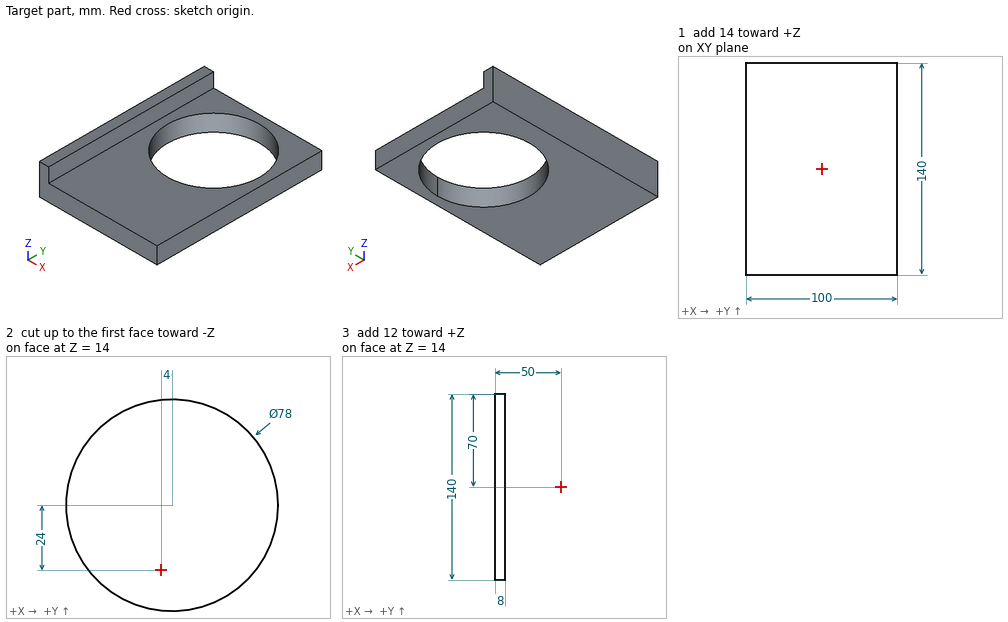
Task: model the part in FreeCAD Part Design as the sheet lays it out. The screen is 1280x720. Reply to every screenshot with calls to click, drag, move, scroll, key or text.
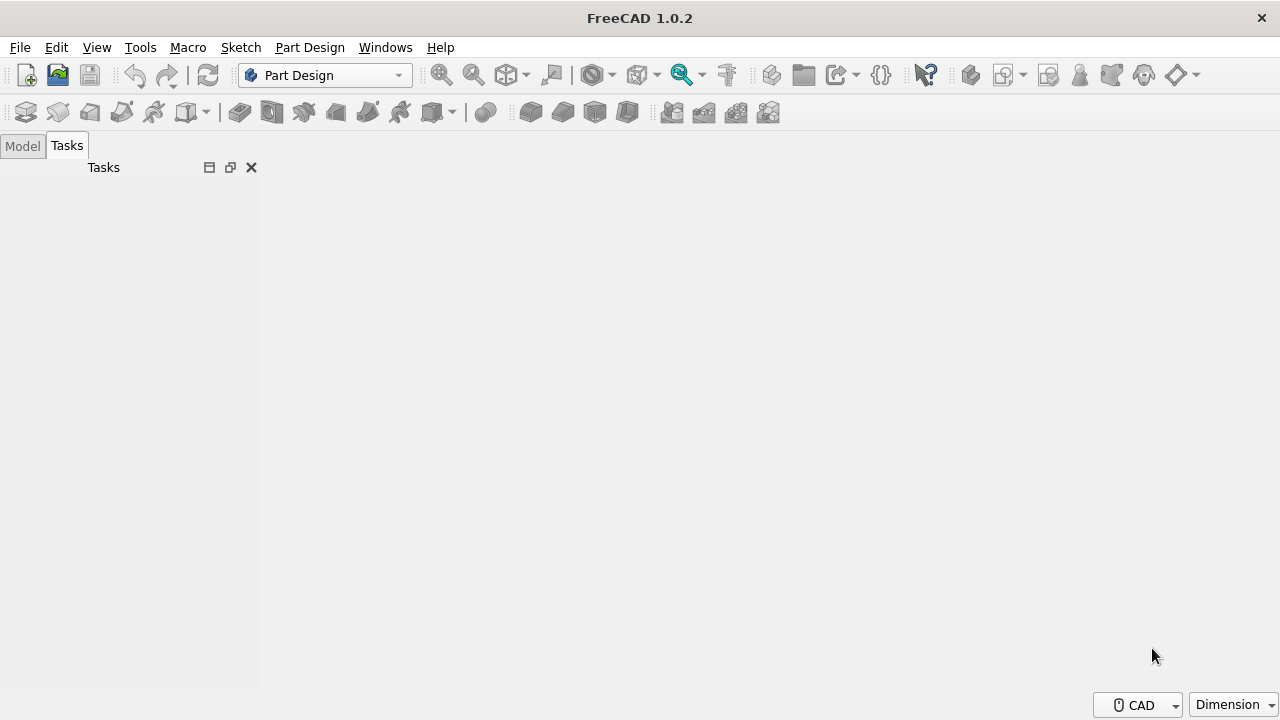
key(ctrl+n)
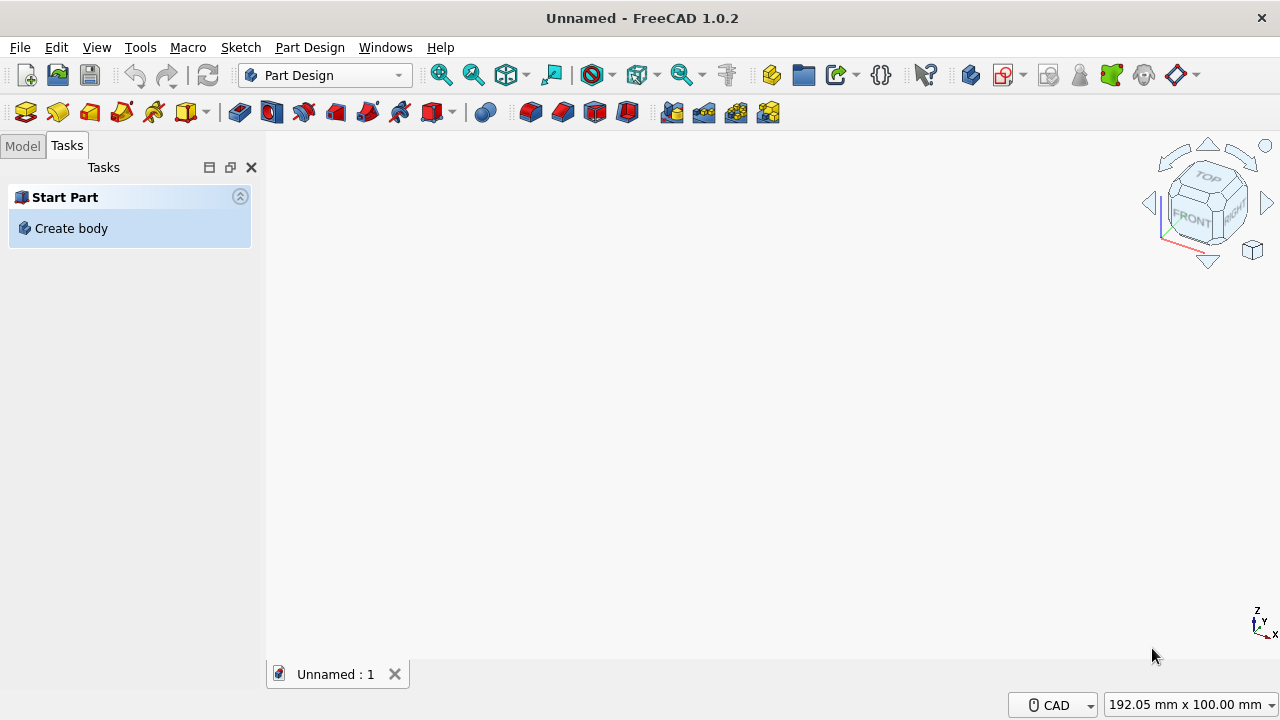
click(1004, 76)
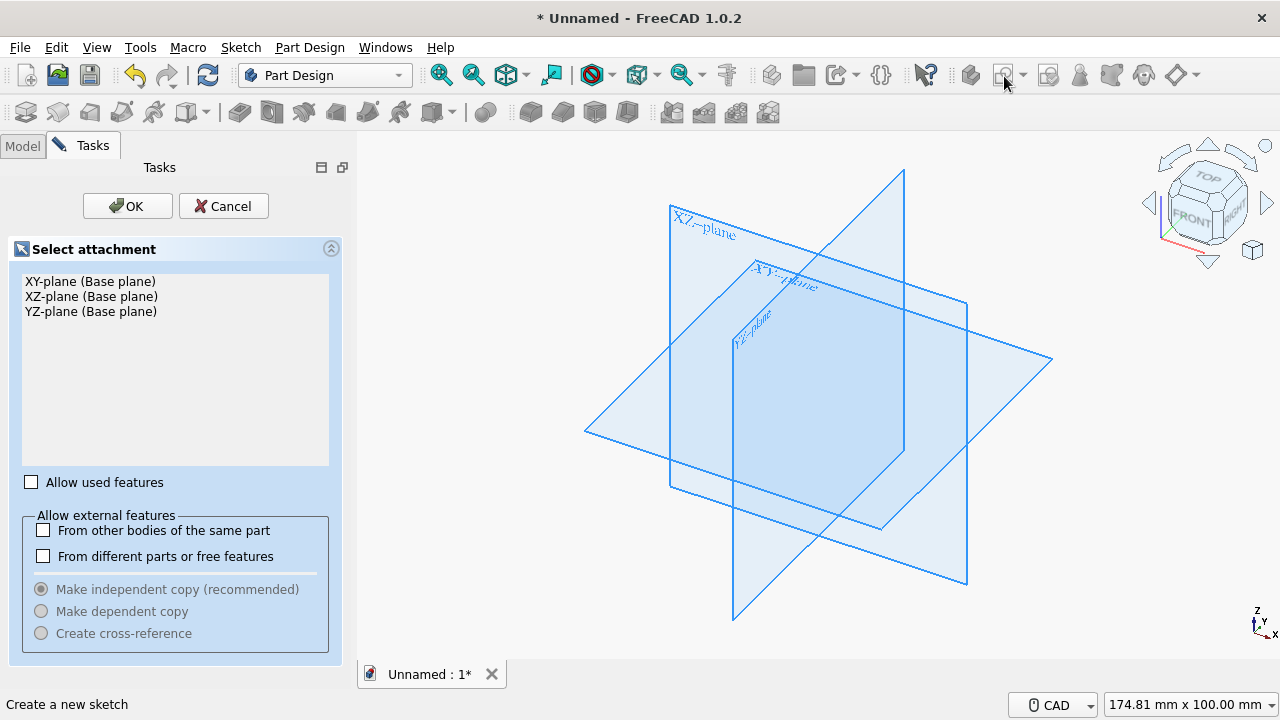
click(82, 282)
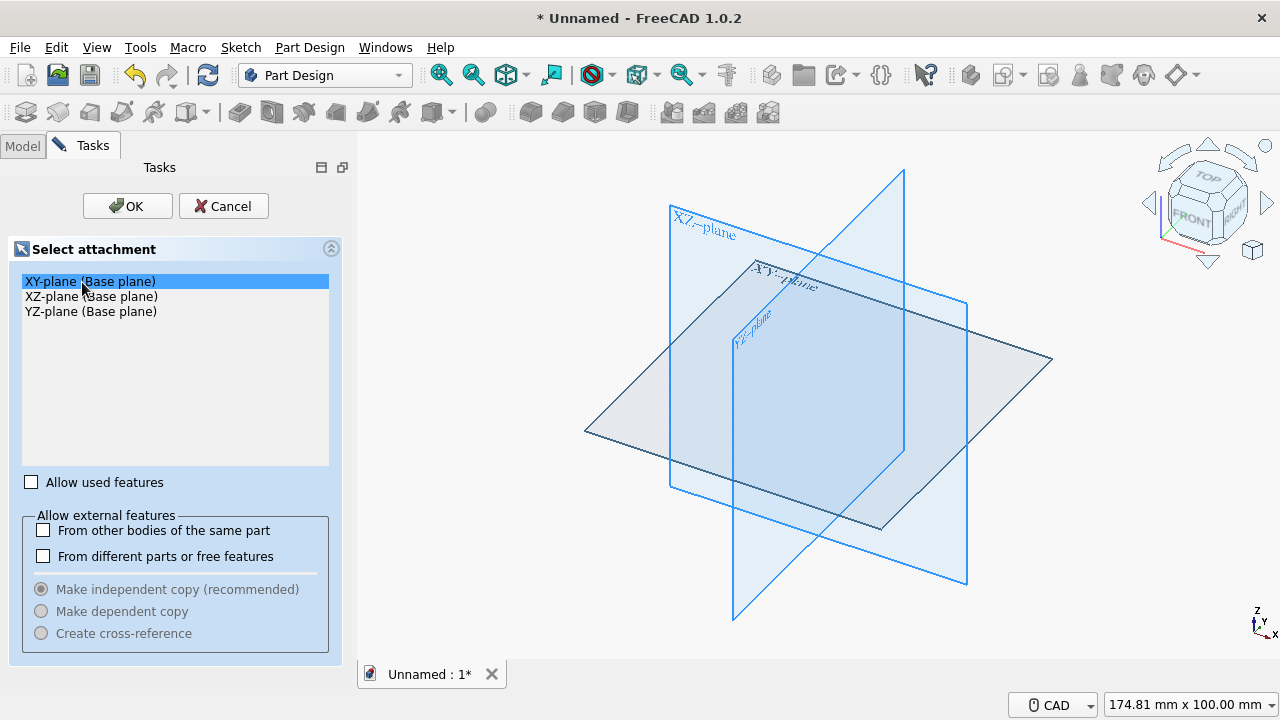
click(128, 206)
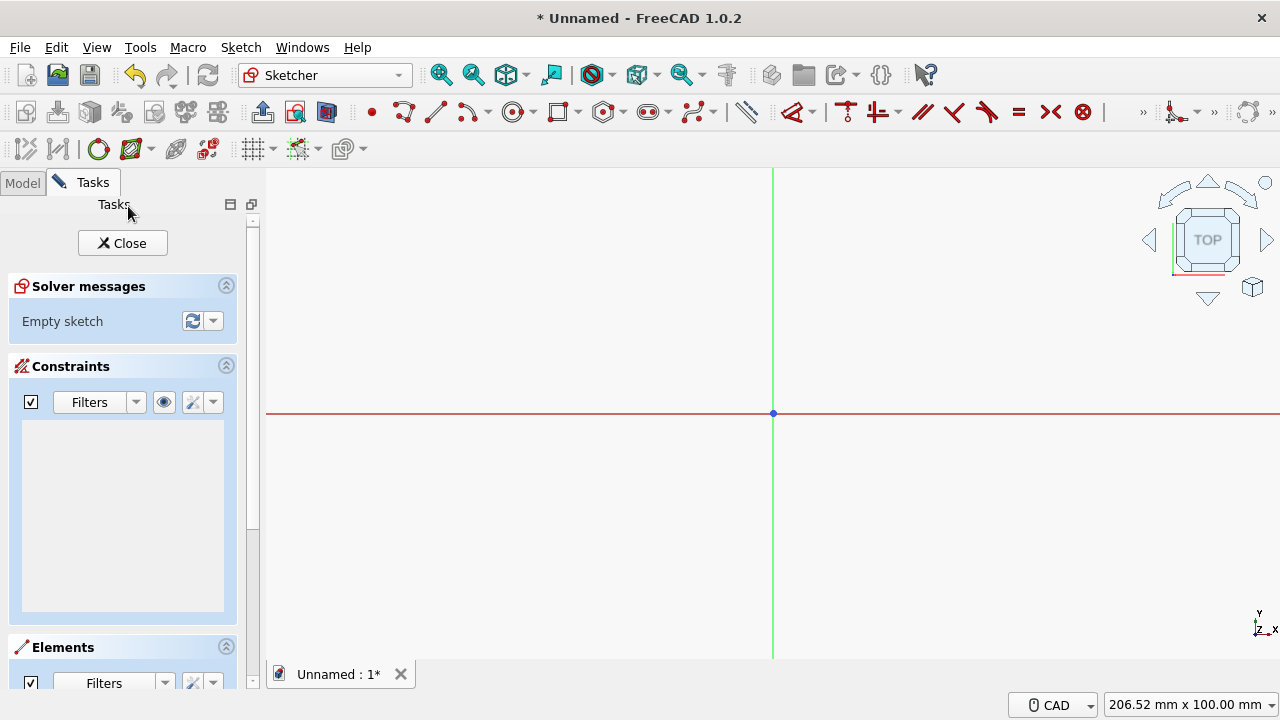
scroll(649, 414, down, 4)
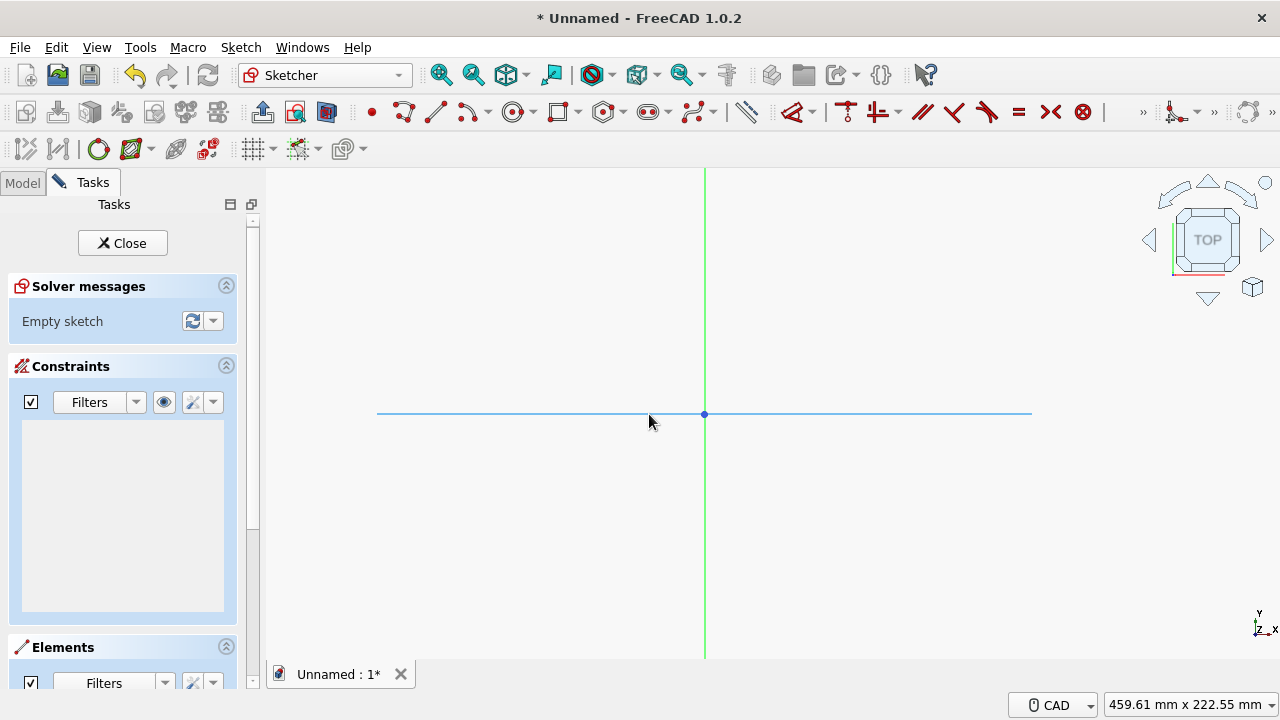
click(580, 112)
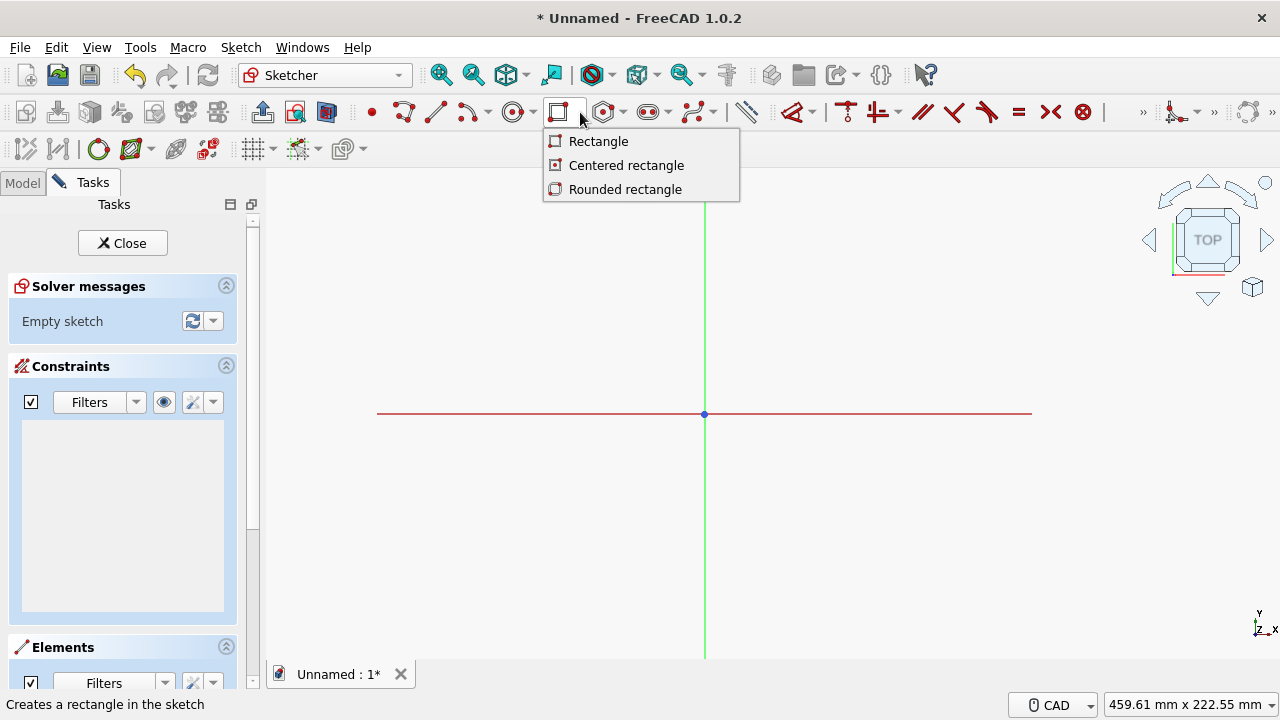
click(642, 165)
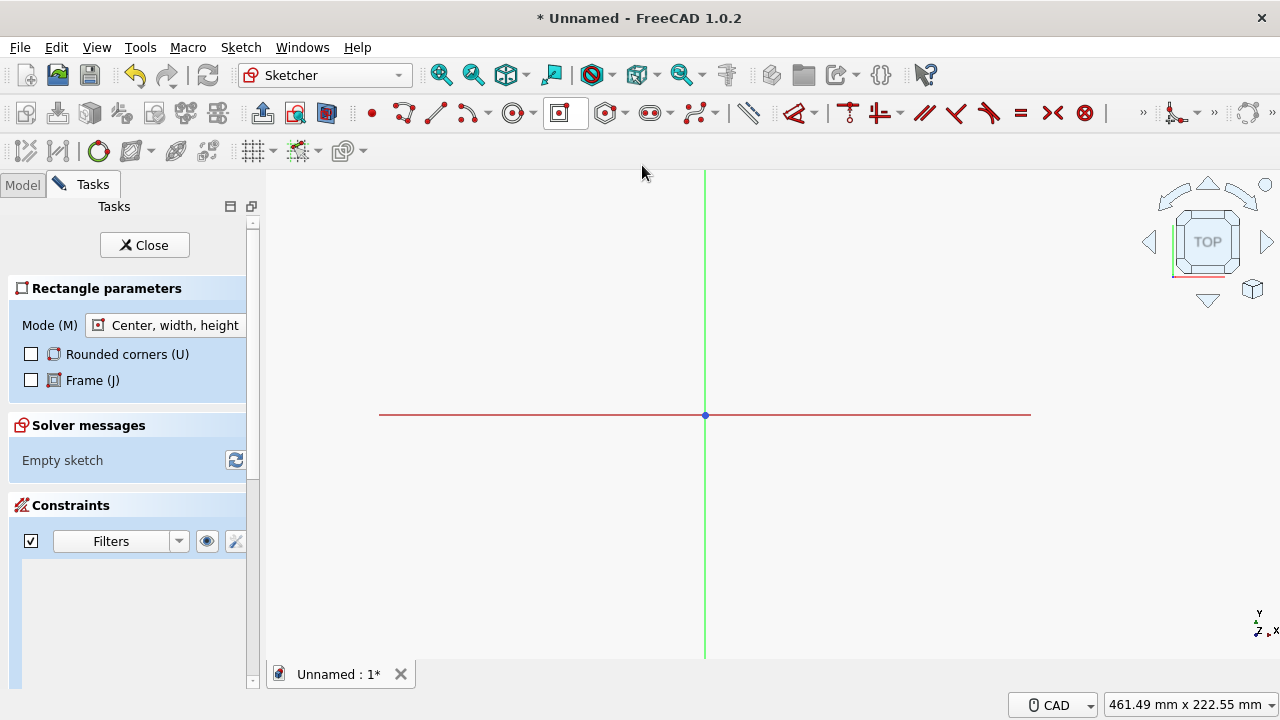
click(705, 415)
move(815, 261)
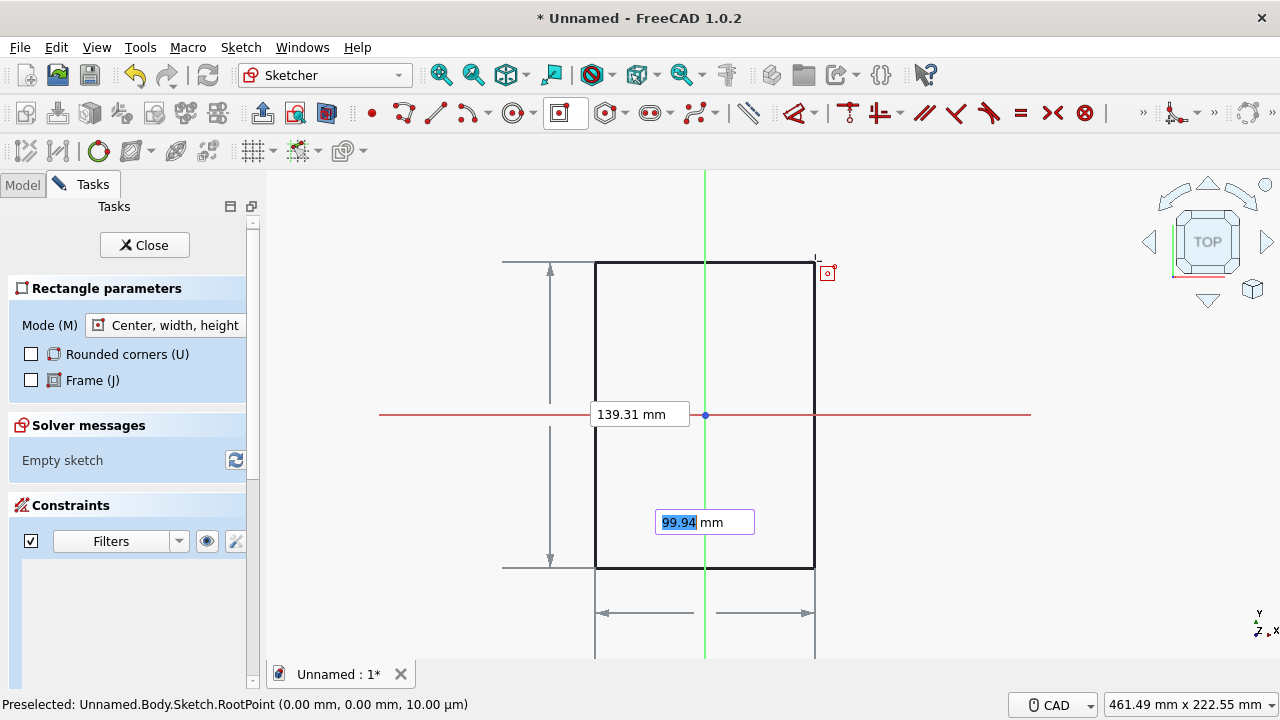
text(100)
key(Tab)
text(140)
key(Return)
key(Escape)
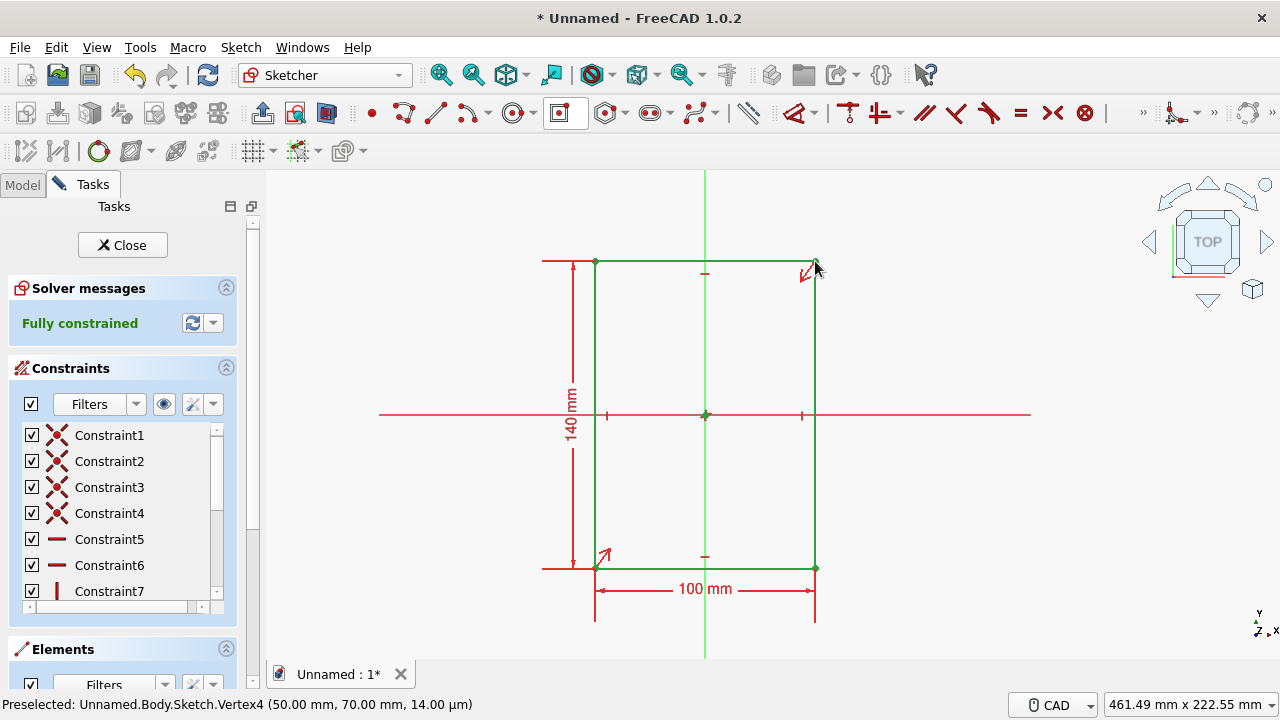
click(123, 245)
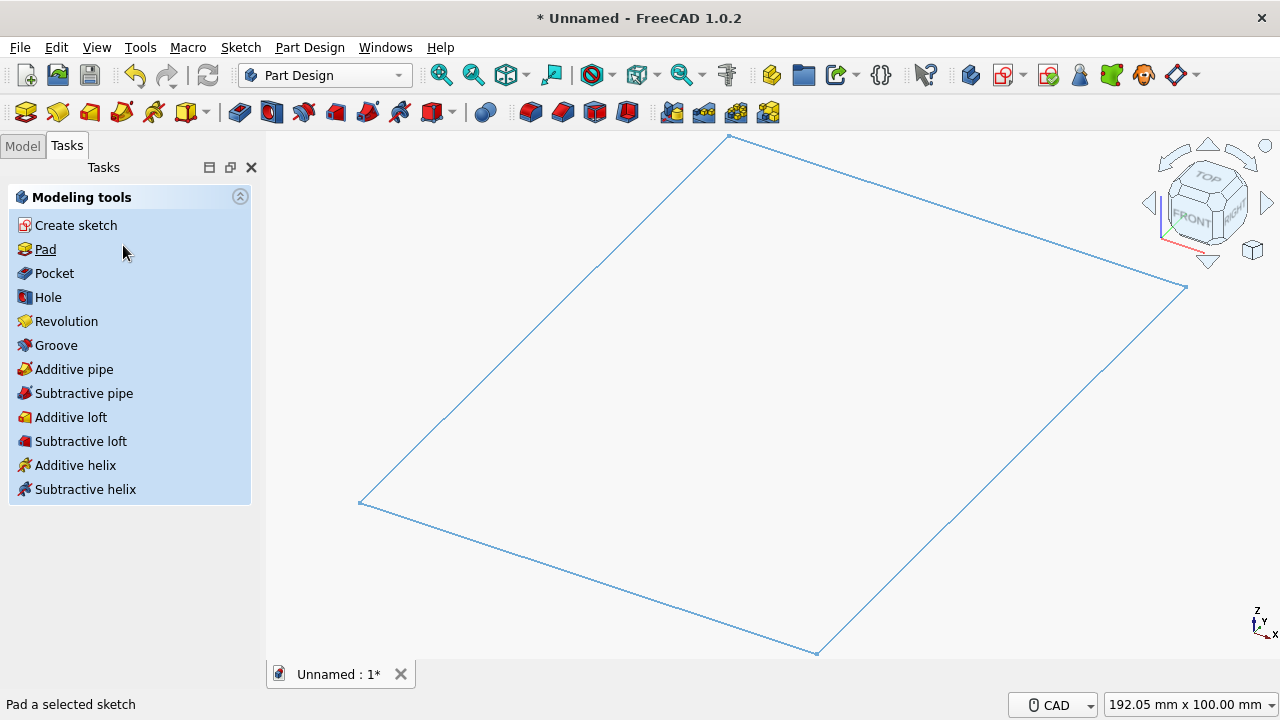
click(26, 112)